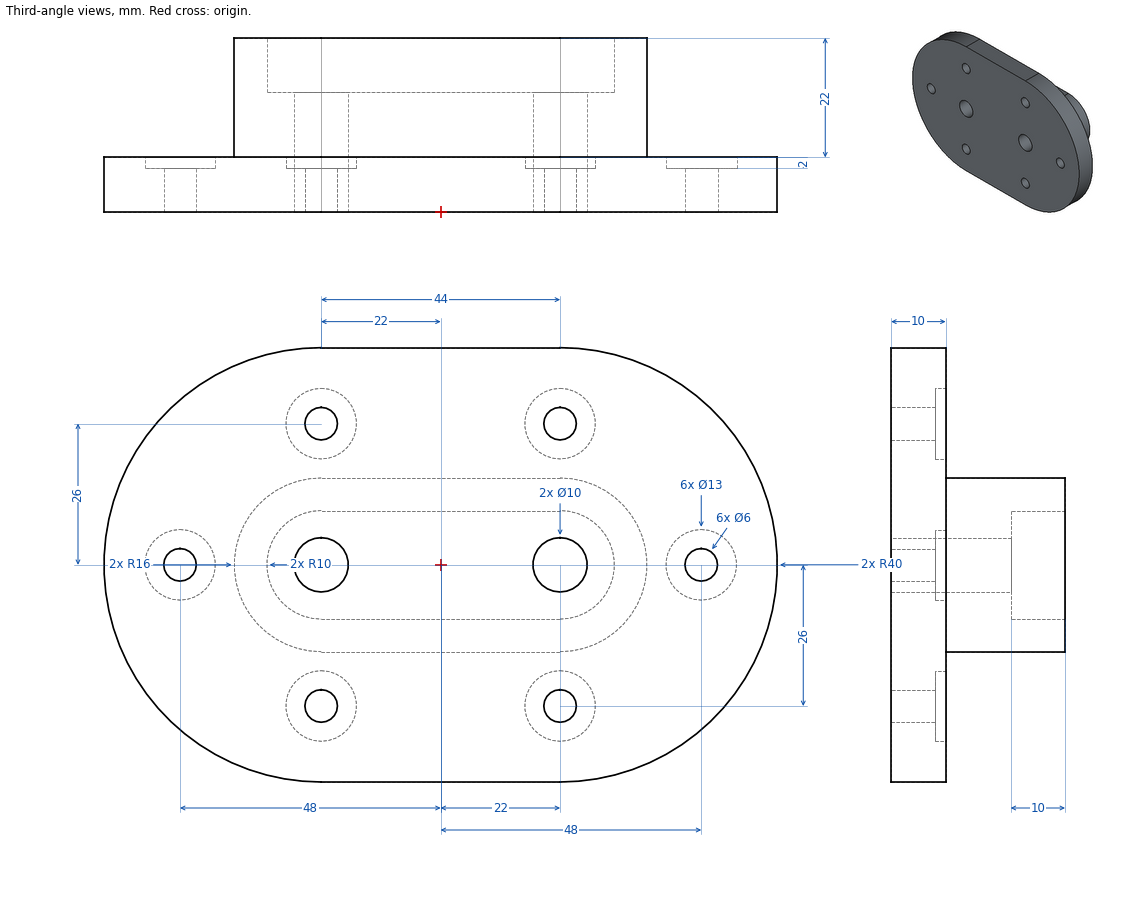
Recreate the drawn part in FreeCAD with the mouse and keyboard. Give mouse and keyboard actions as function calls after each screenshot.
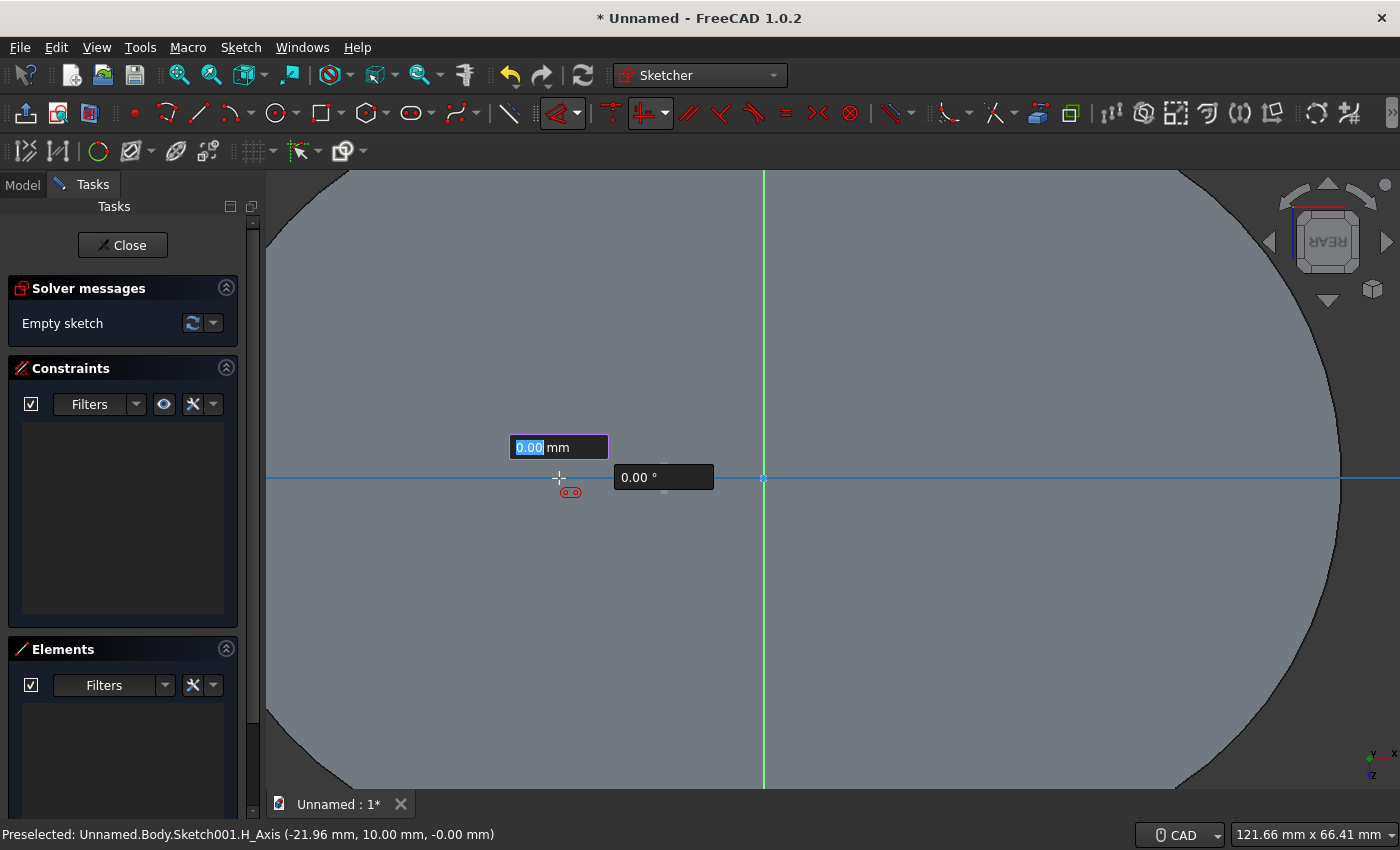
click(969, 469)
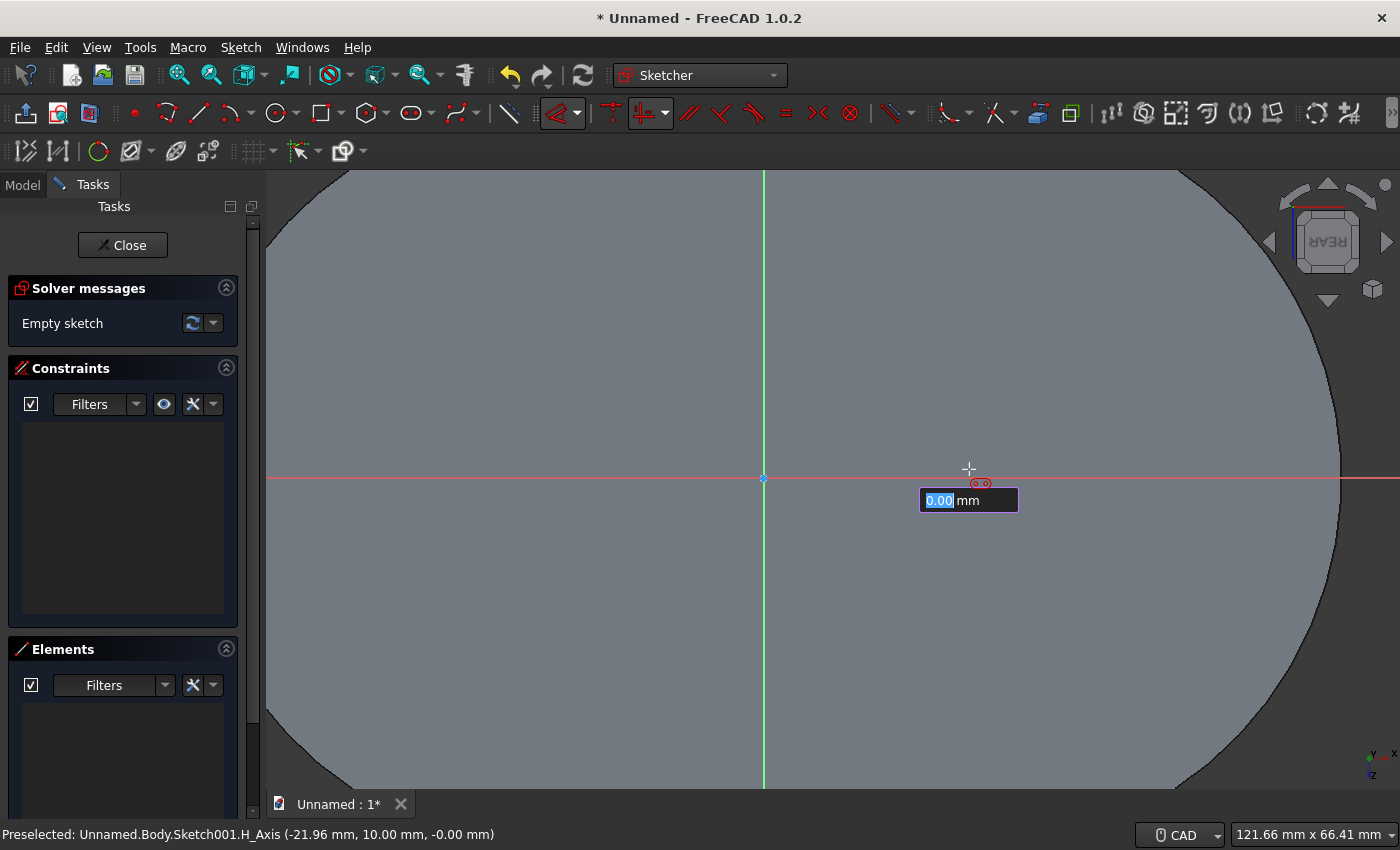
click(825, 329)
key(Escape)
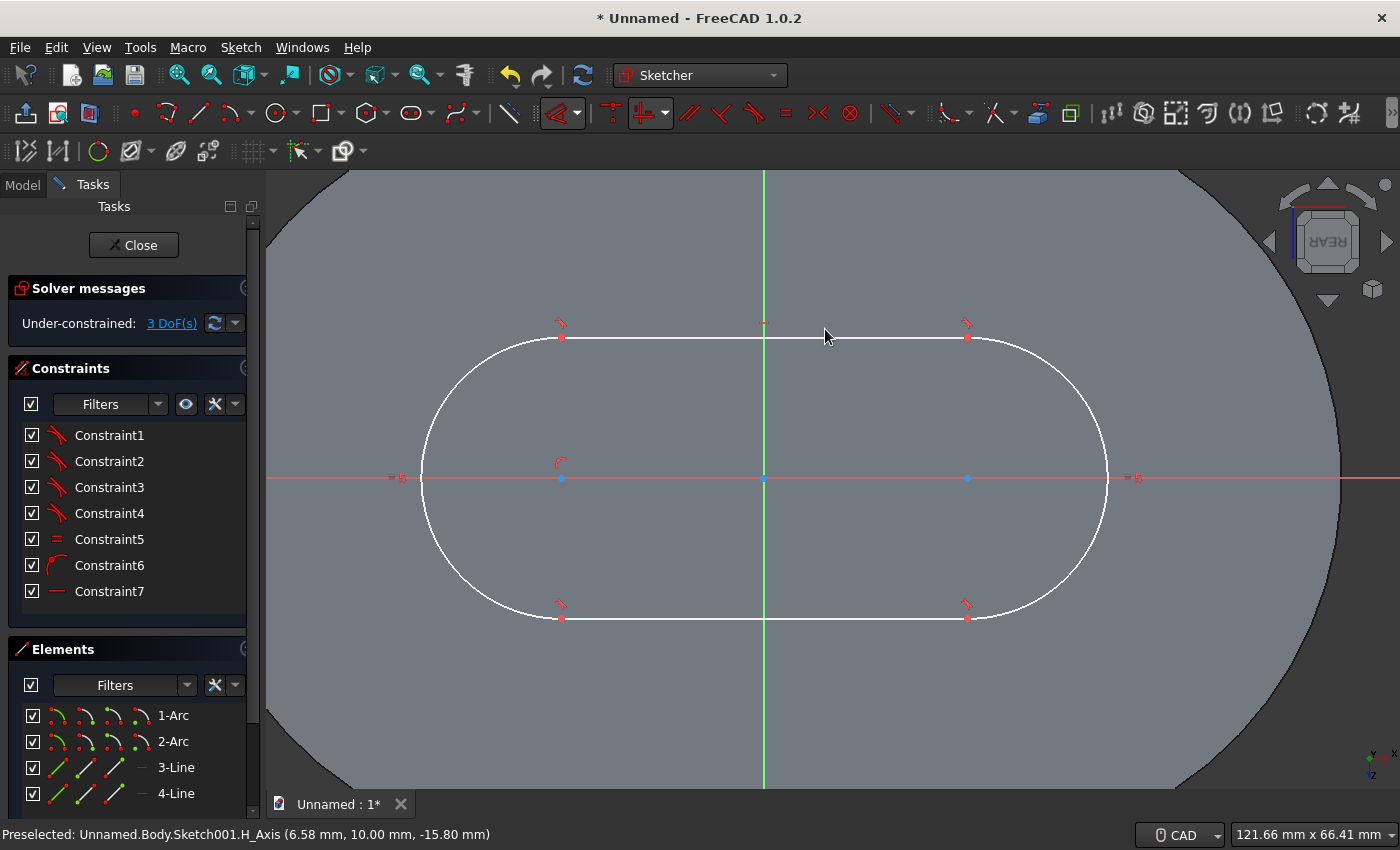
click(448, 396)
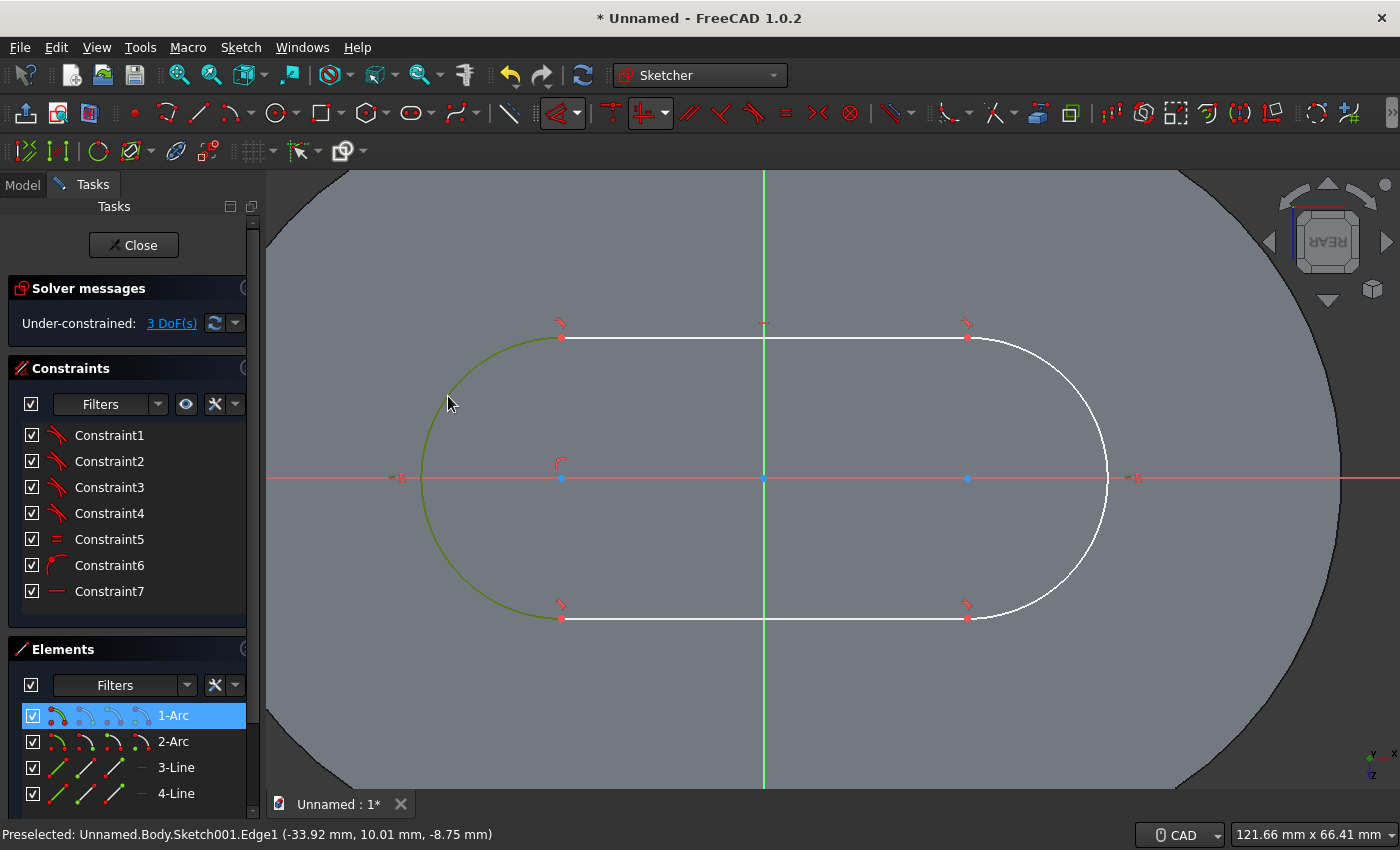
click(580, 114)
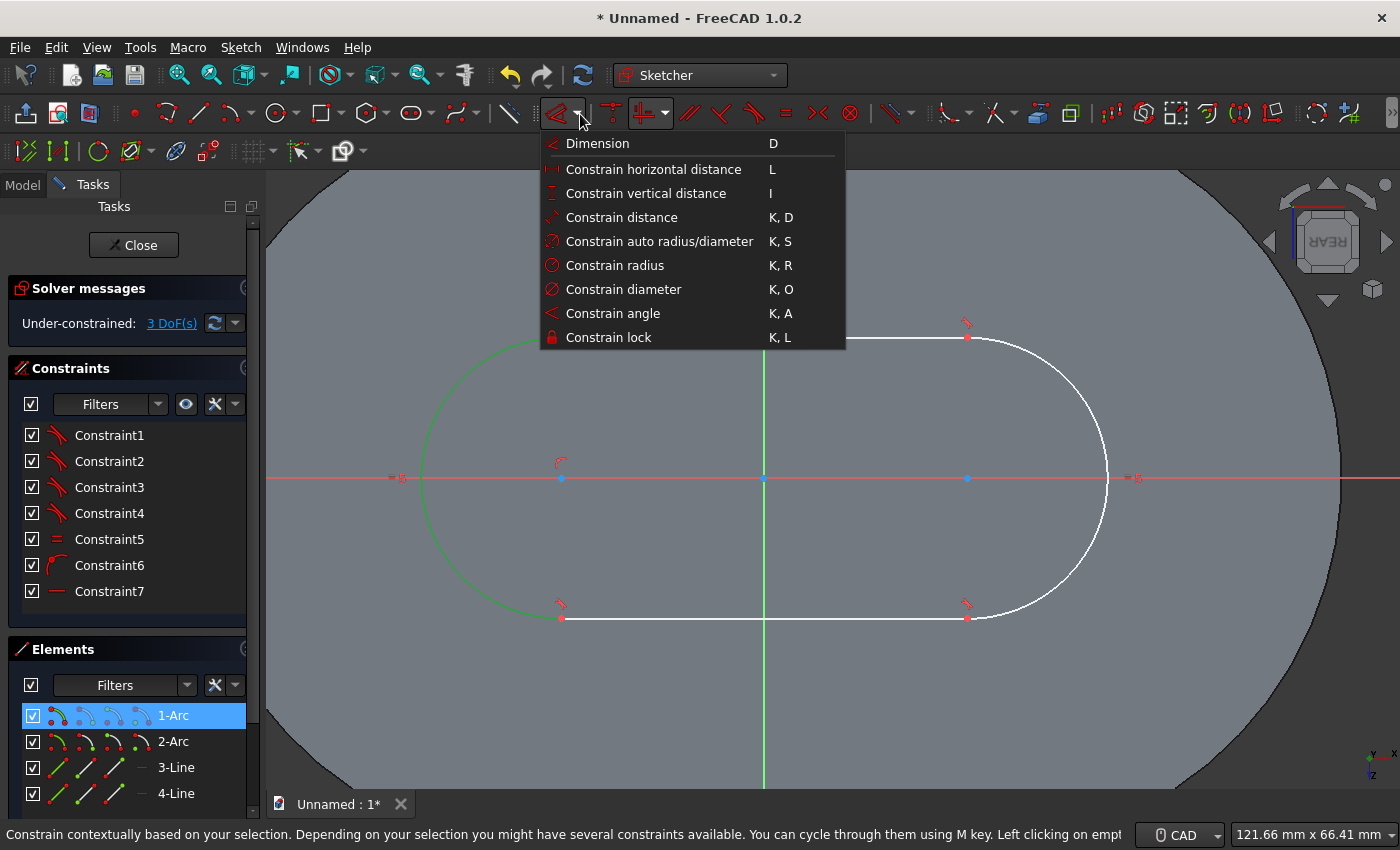
click(693, 265)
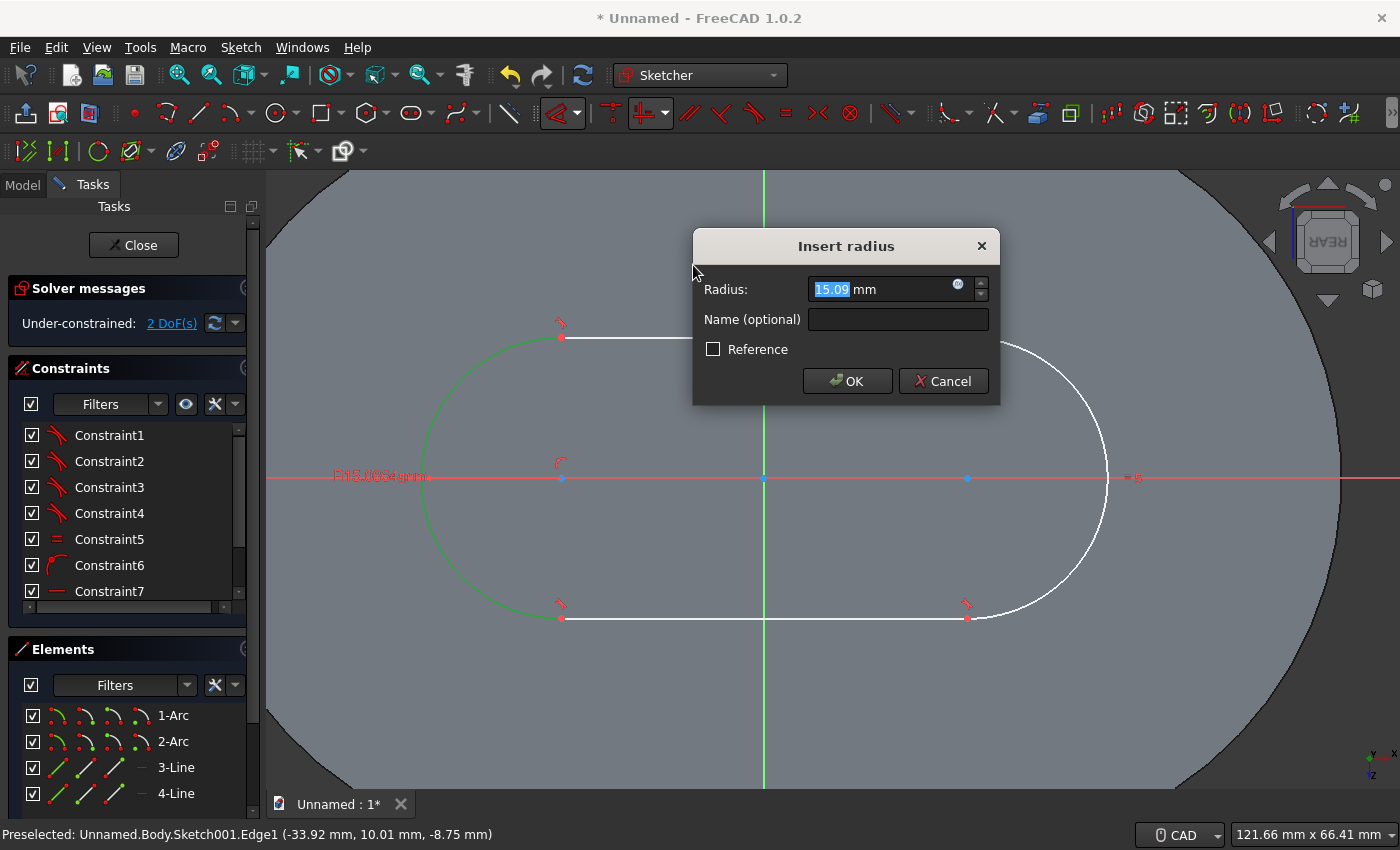
text(16)
key(Return)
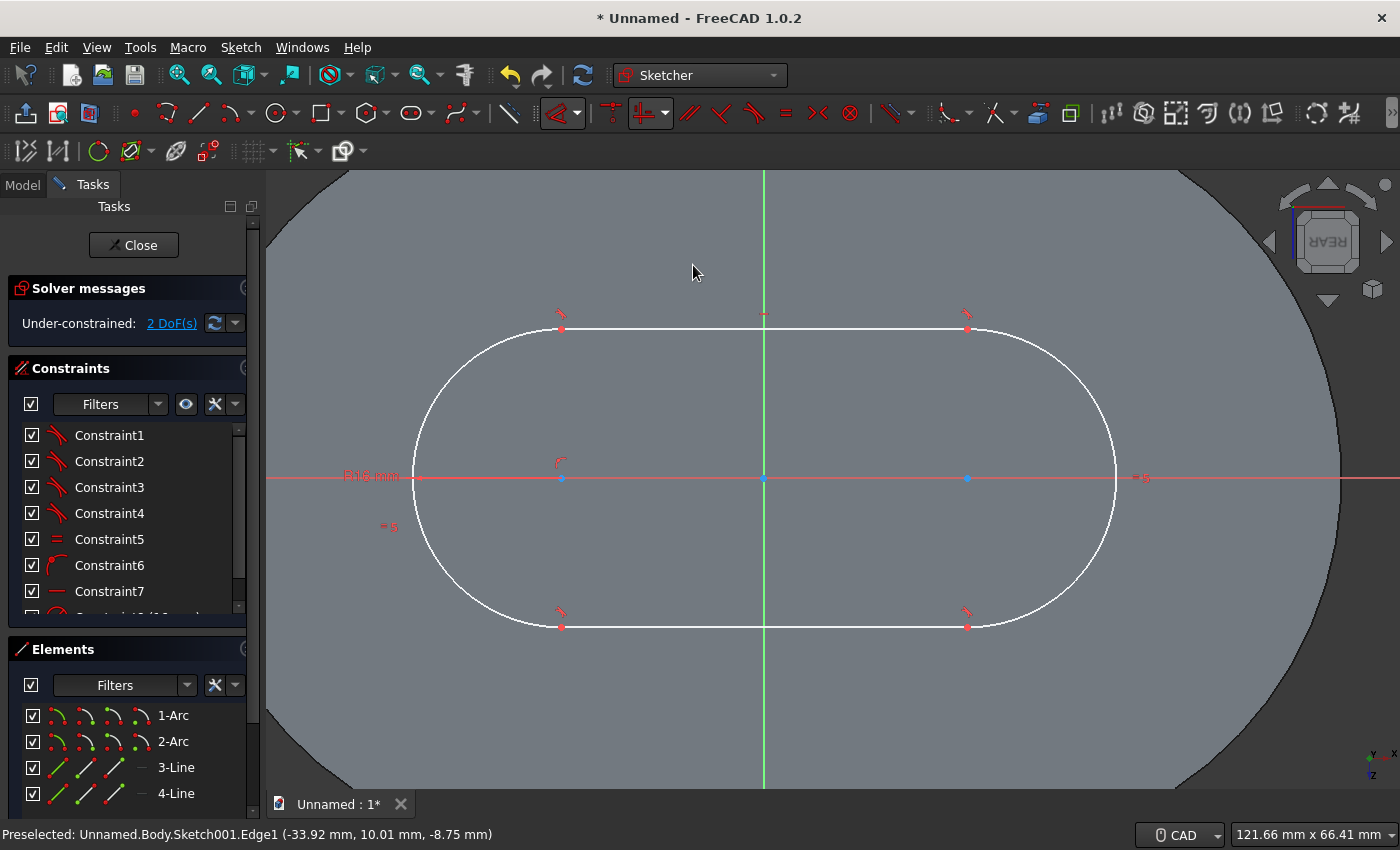
click(684, 329)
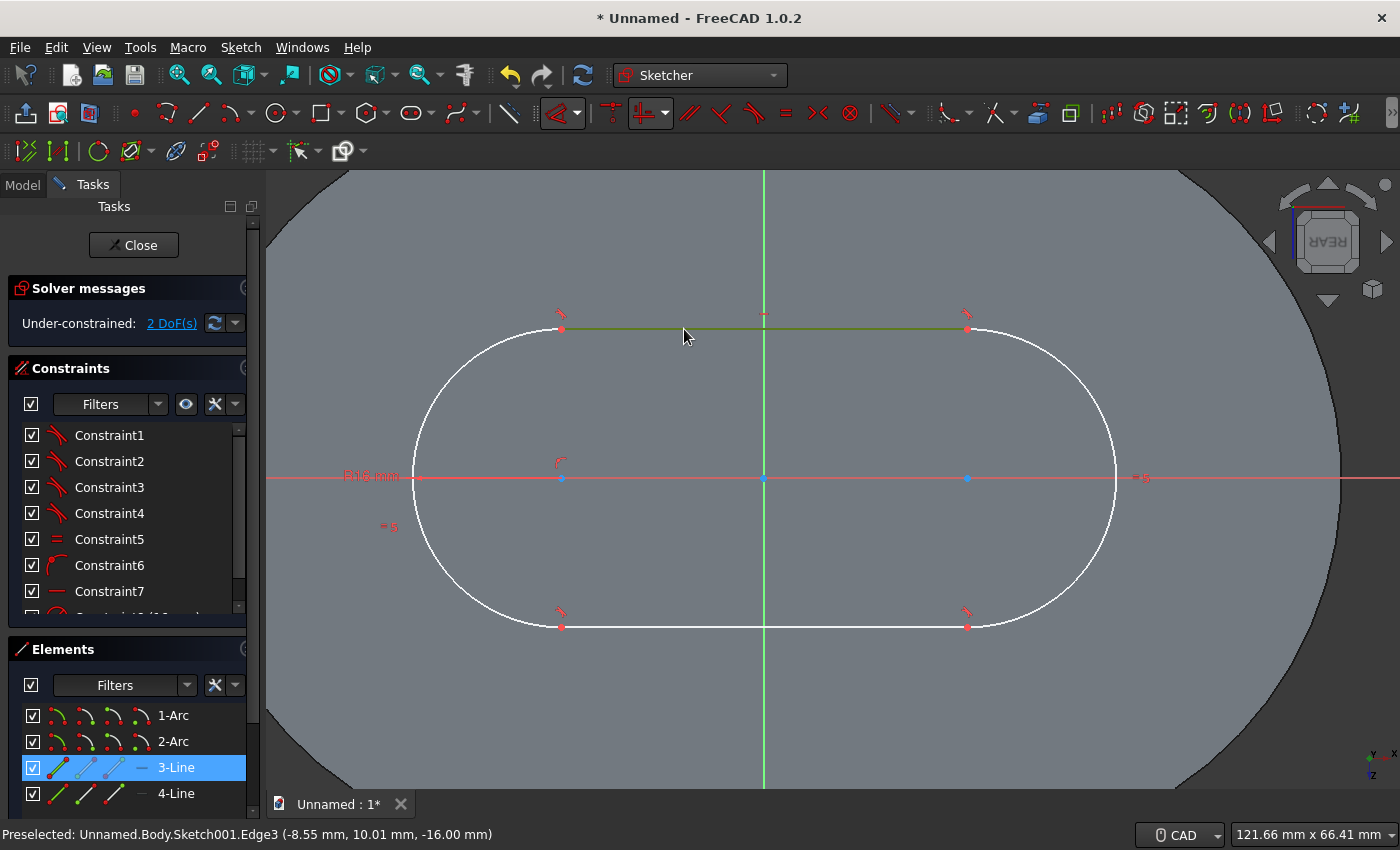
click(580, 114)